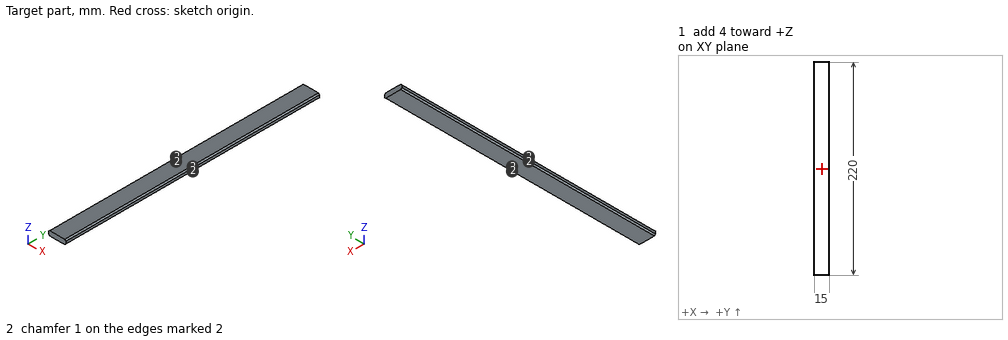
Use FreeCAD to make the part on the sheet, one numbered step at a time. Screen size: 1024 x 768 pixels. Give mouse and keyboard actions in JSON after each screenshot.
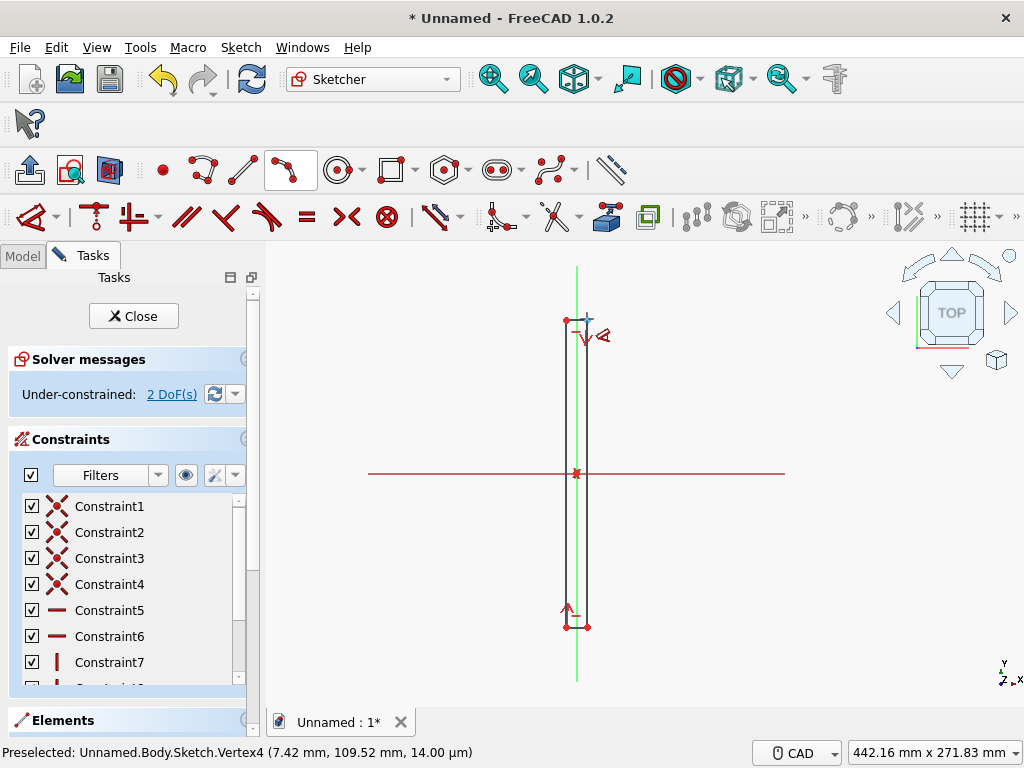
{"action": "scroll", "coordinate": [575, 628], "scroll_direction": "up", "scroll_amount": 4}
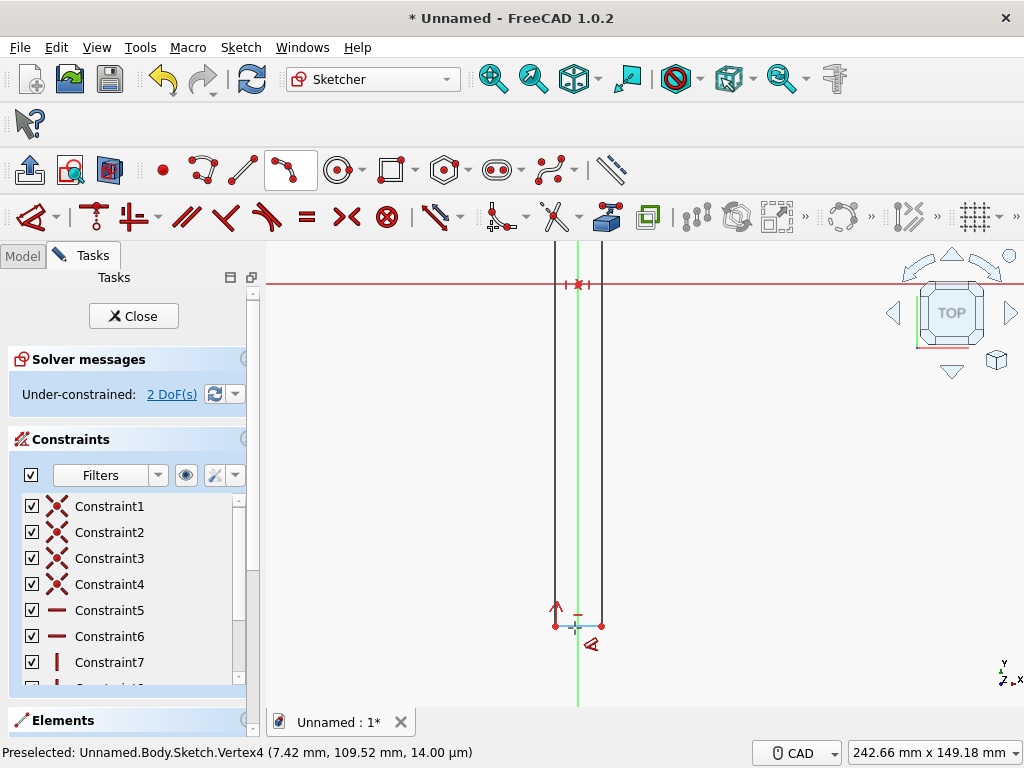
{"action": "left_click", "coordinate": [574, 626]}
{"action": "left_click", "coordinate": [562, 660]}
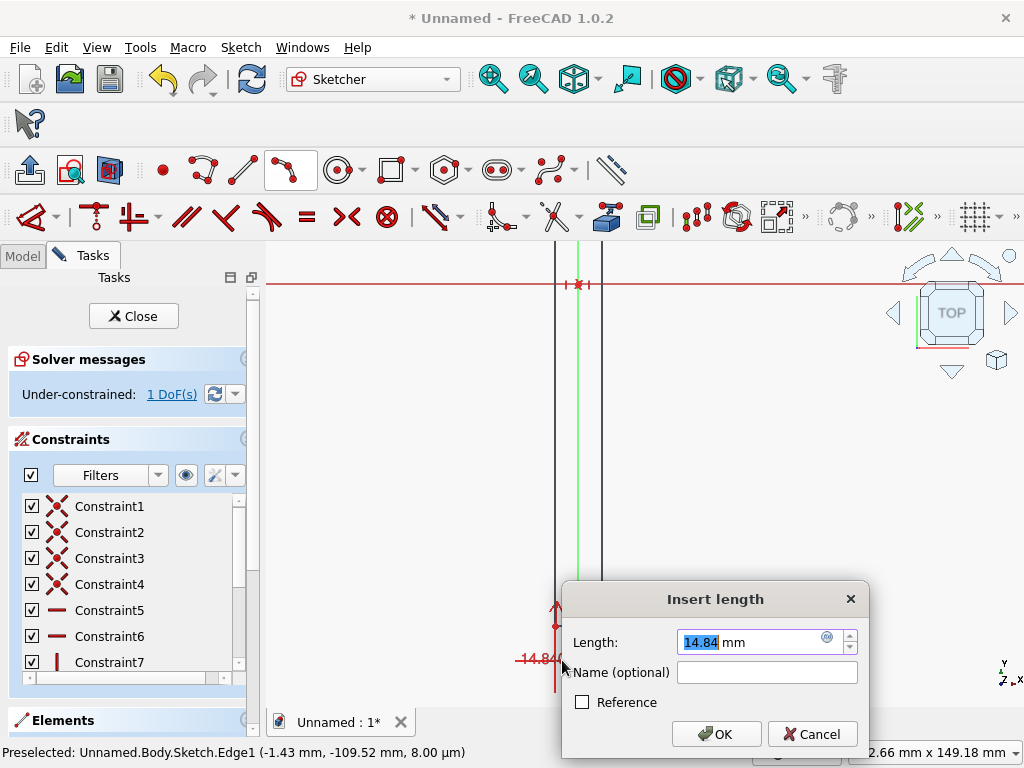
{"action": "type", "text": "15"}
{"action": "key", "text": "Return"}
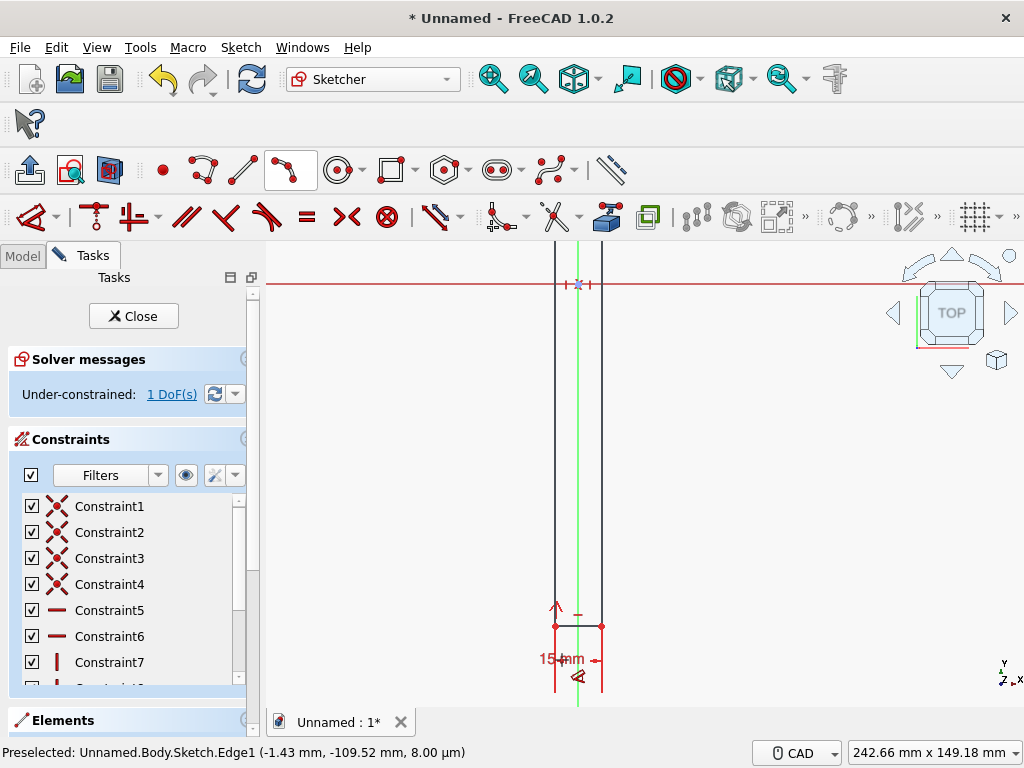
{"action": "left_click", "coordinate": [602, 421]}
{"action": "left_click", "coordinate": [636, 448]}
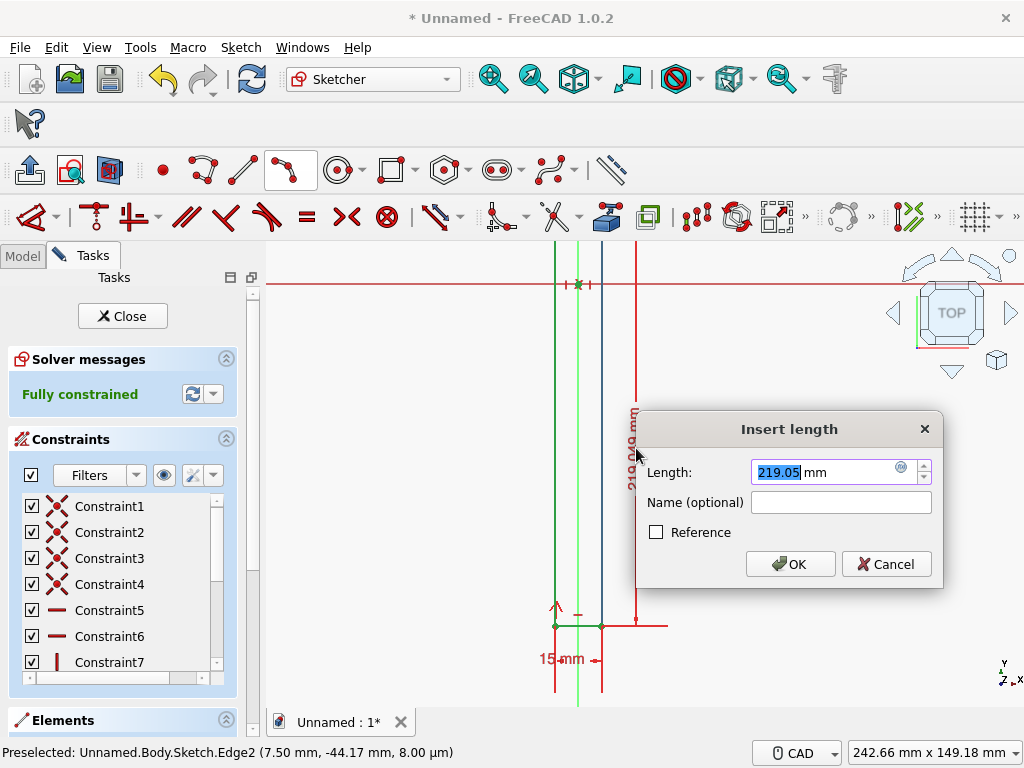
{"action": "type", "text": "220"}
{"action": "key", "text": "Return"}
{"action": "key", "text": "Escape"}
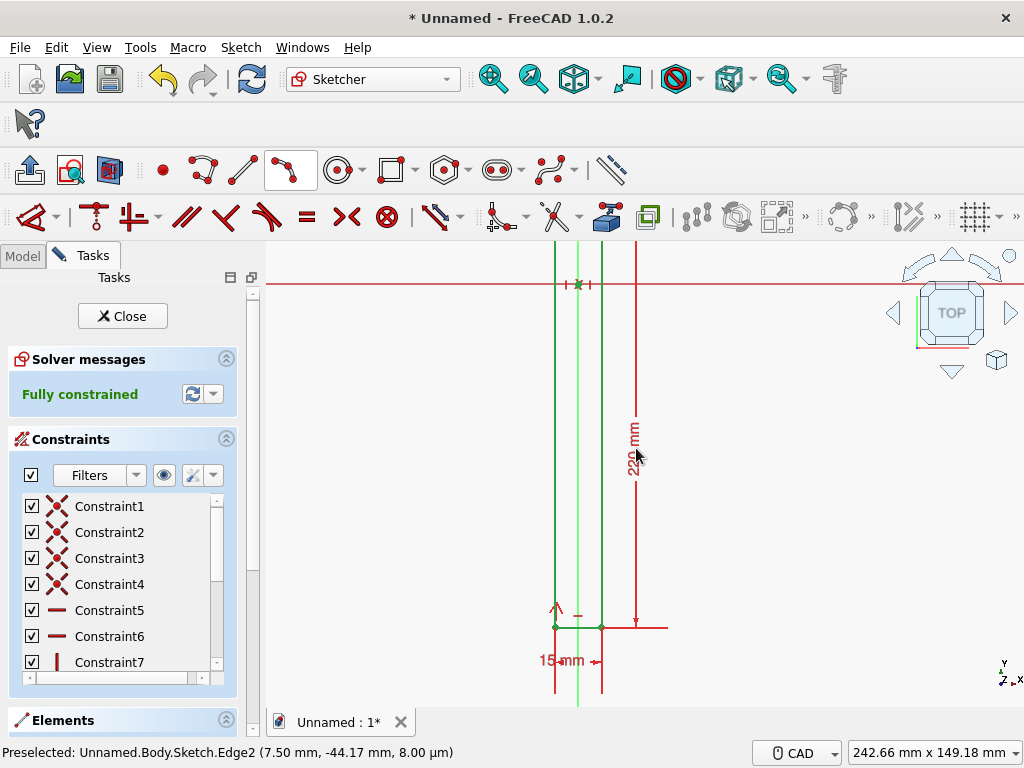
{"action": "left_click", "coordinate": [123, 316]}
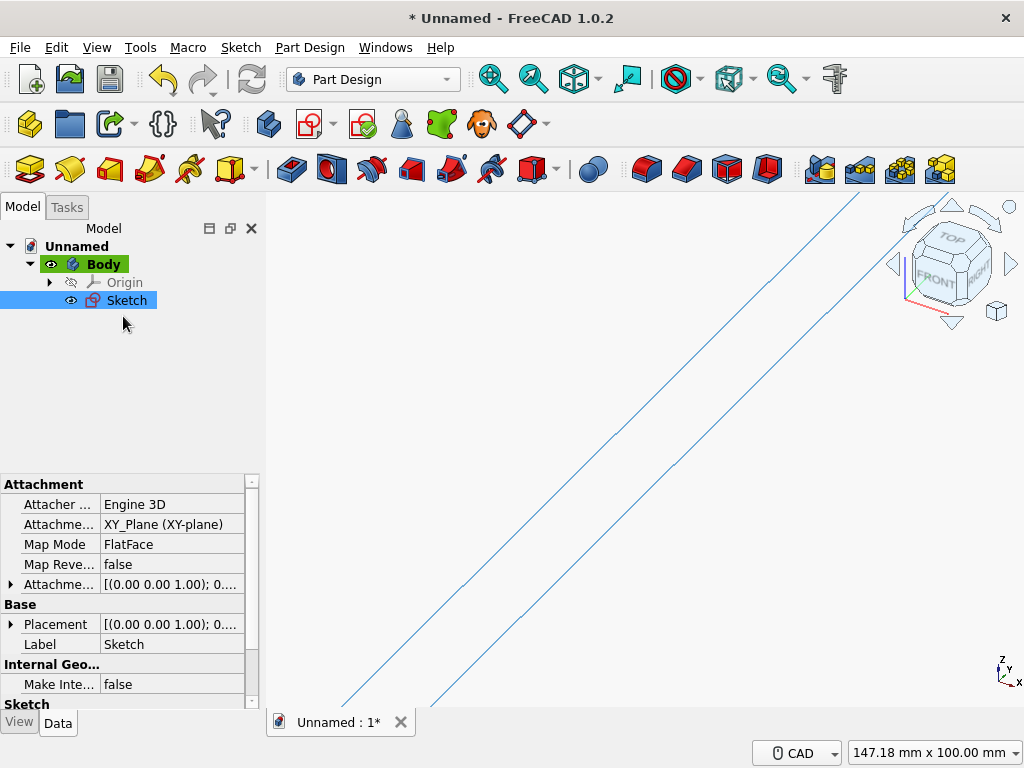
{"action": "left_click", "coordinate": [30, 170]}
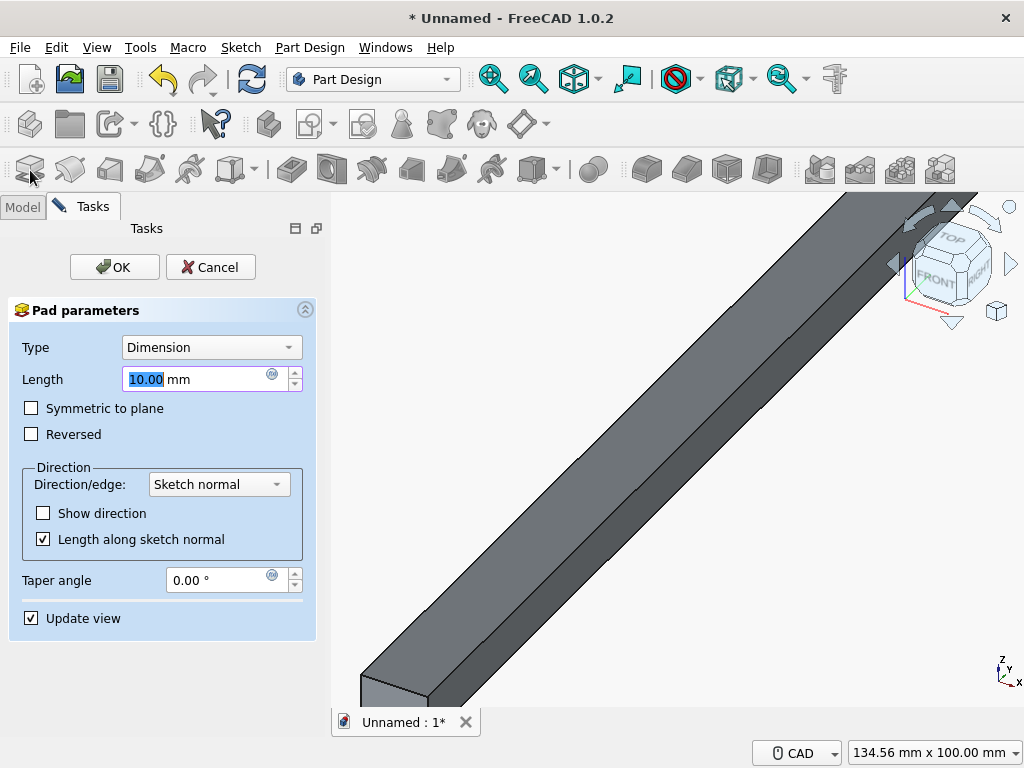
{"action": "type", "text": "4"}
{"action": "key", "text": "Tab"}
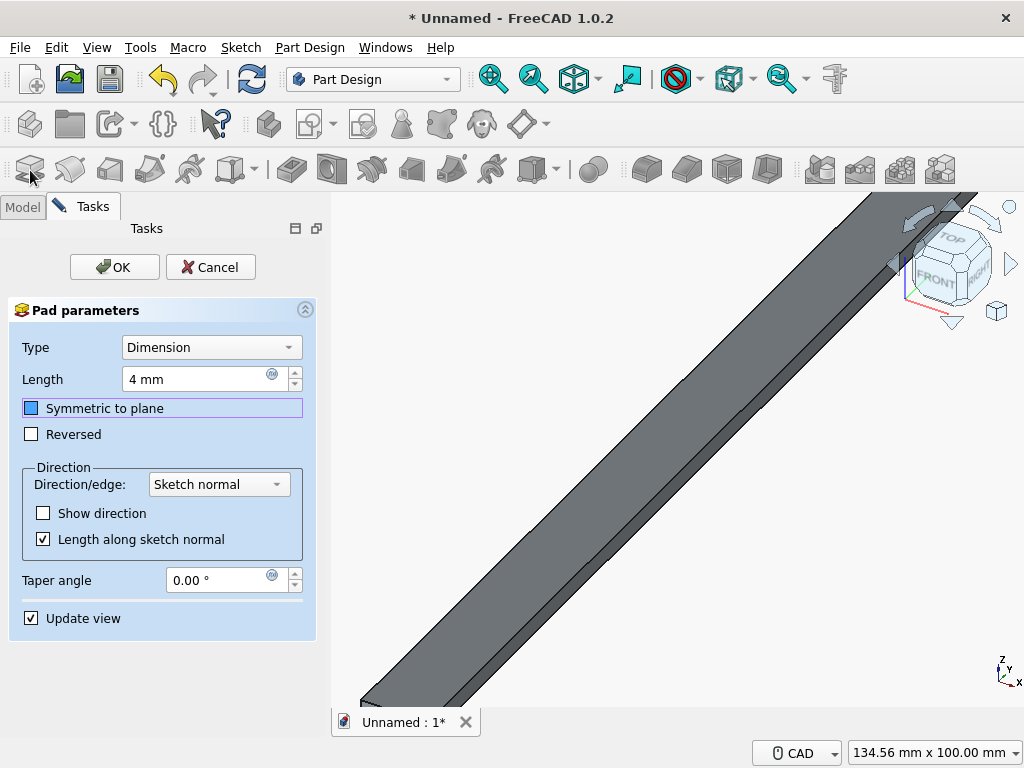
{"action": "left_click", "coordinate": [115, 267]}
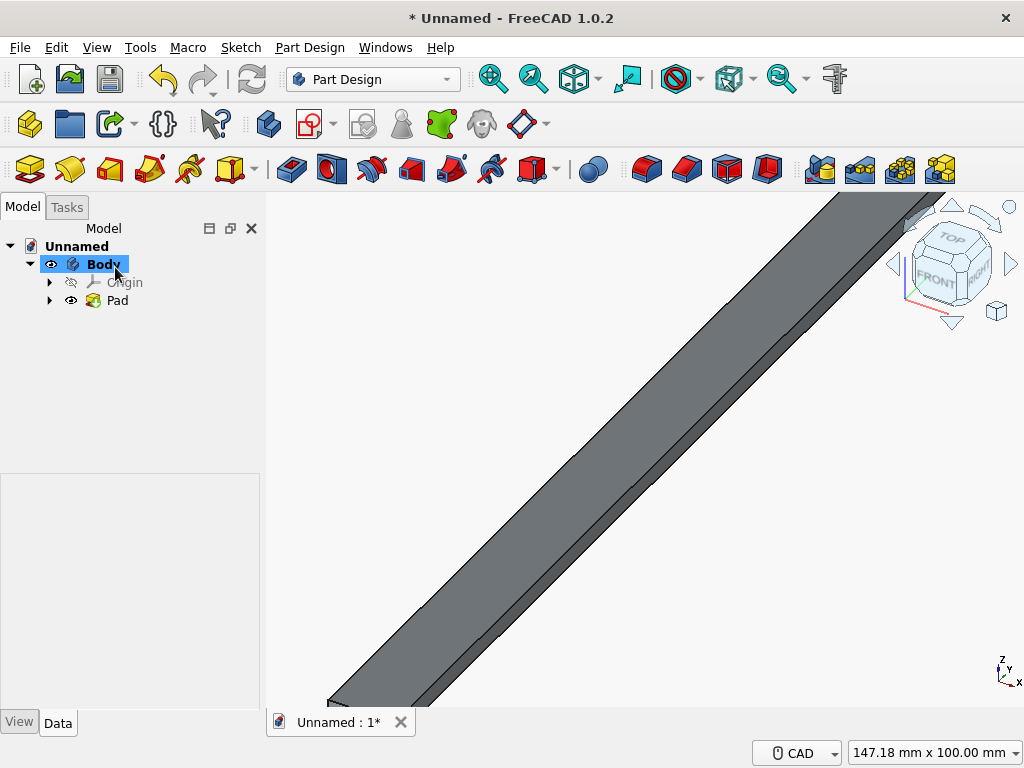
{"action": "left_click", "coordinate": [494, 80]}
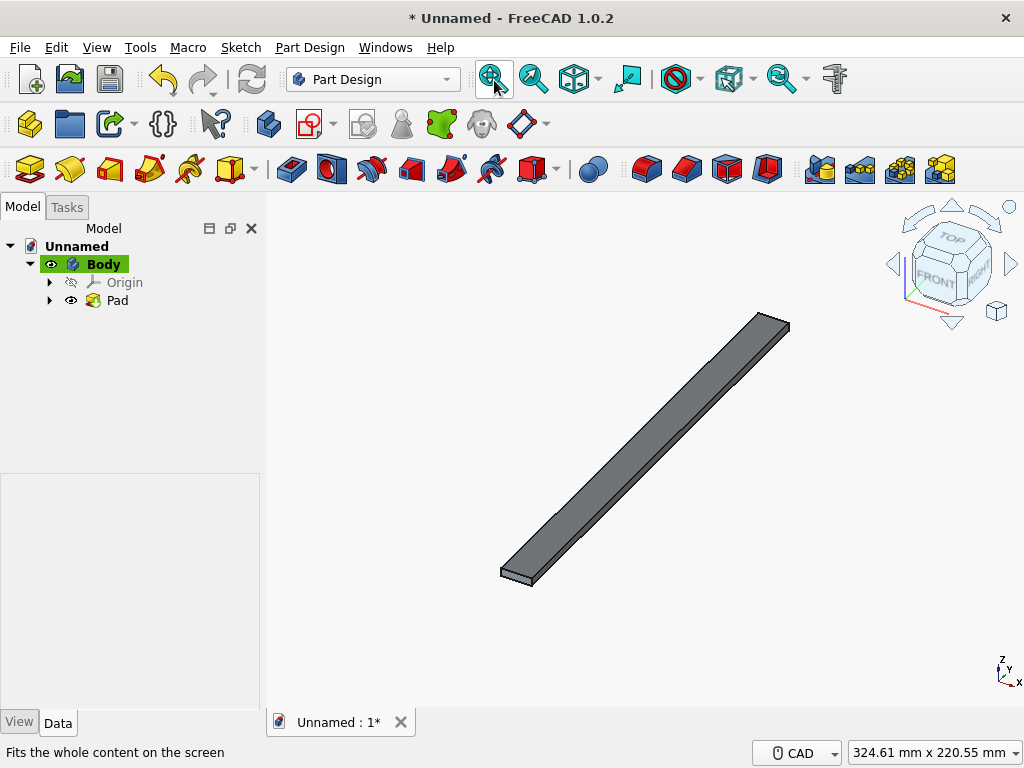
{"action": "left_click", "coordinate": [660, 450]}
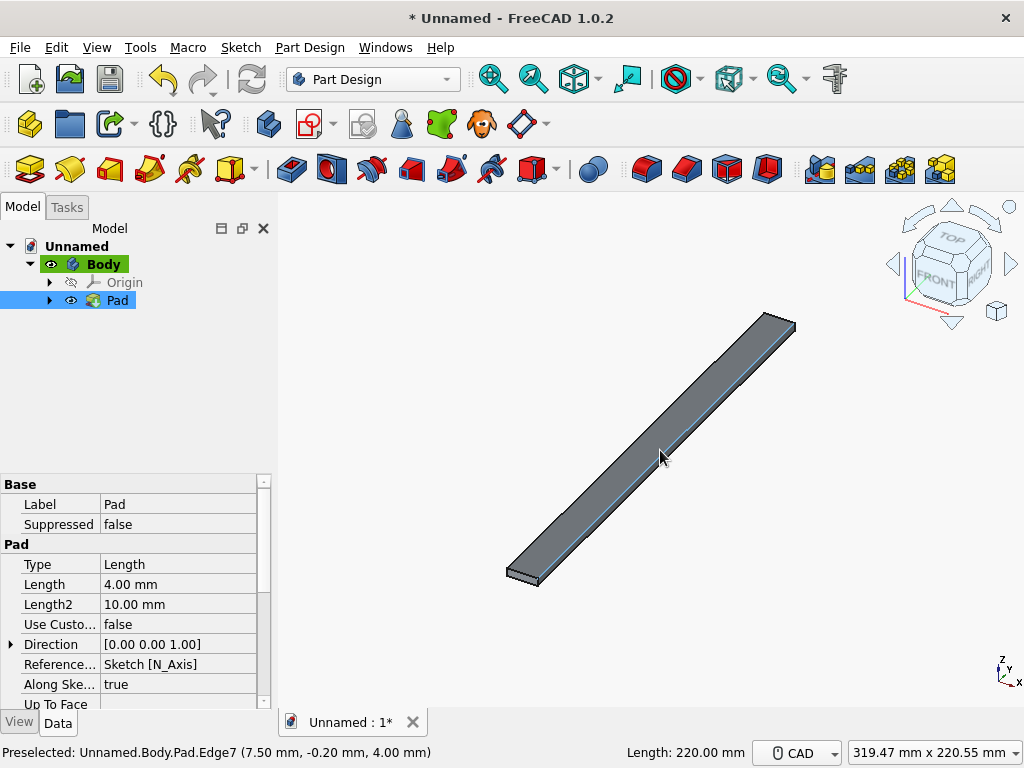
{"action": "key", "text": "0"}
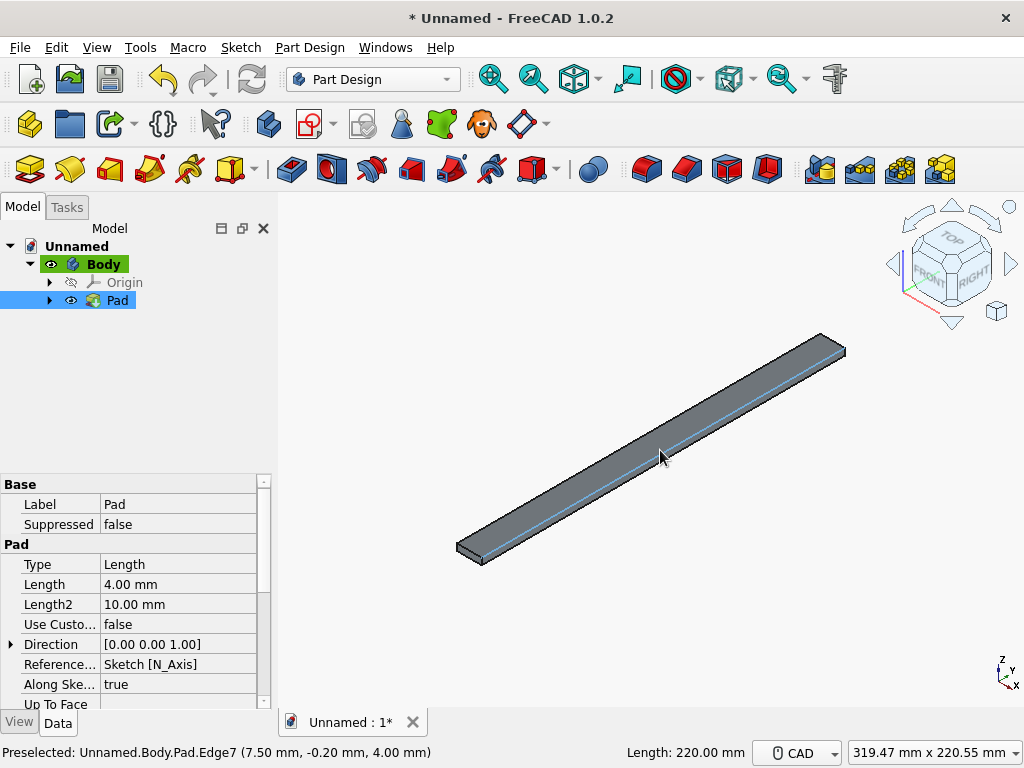
{"action": "key", "text": "2"}